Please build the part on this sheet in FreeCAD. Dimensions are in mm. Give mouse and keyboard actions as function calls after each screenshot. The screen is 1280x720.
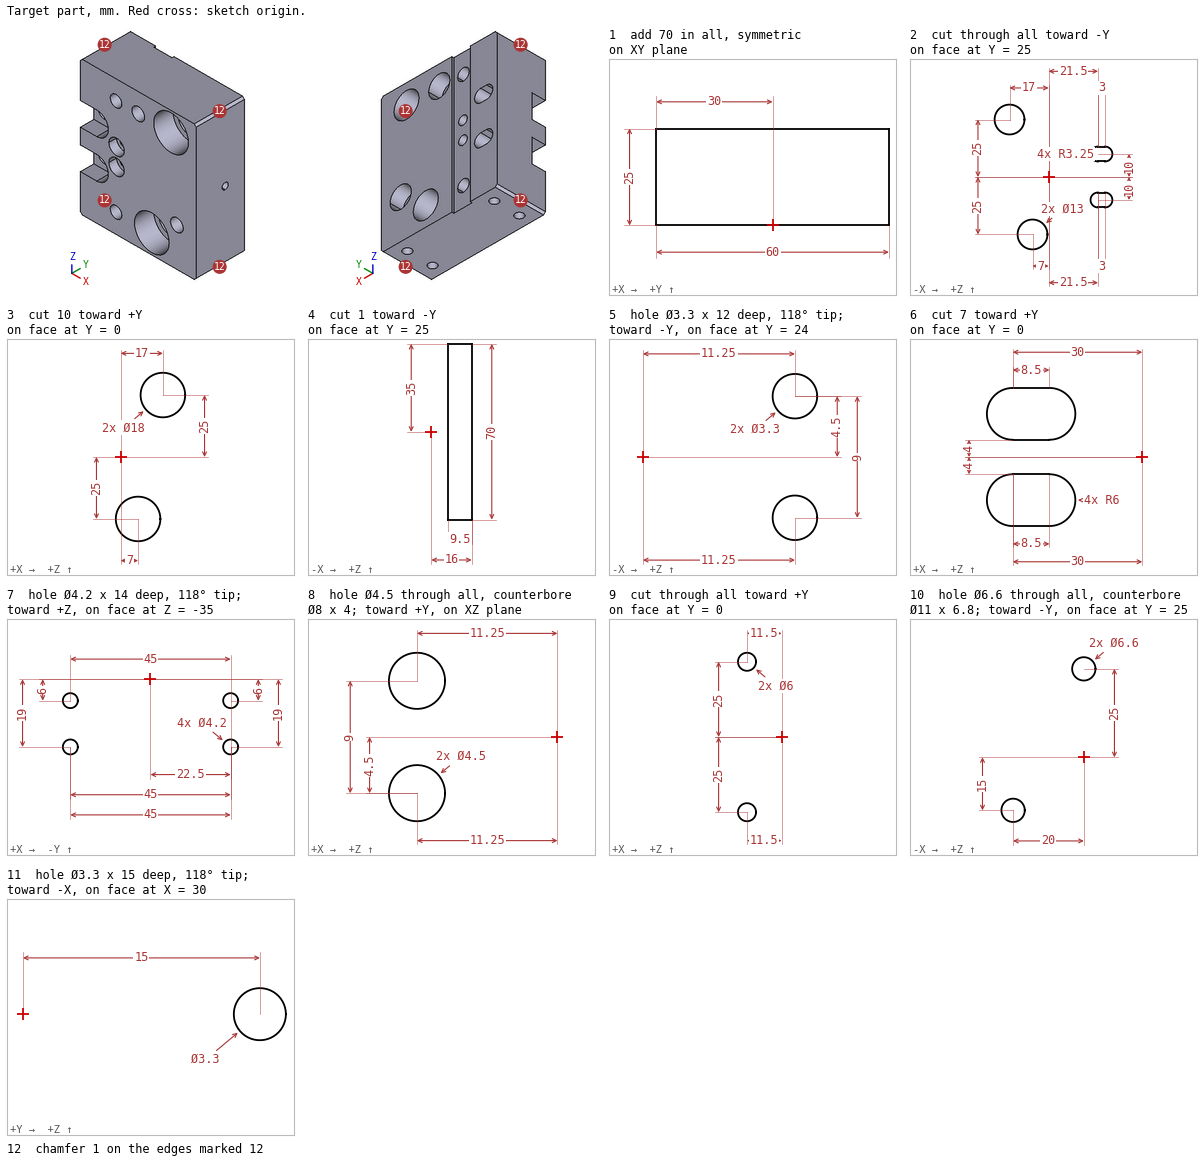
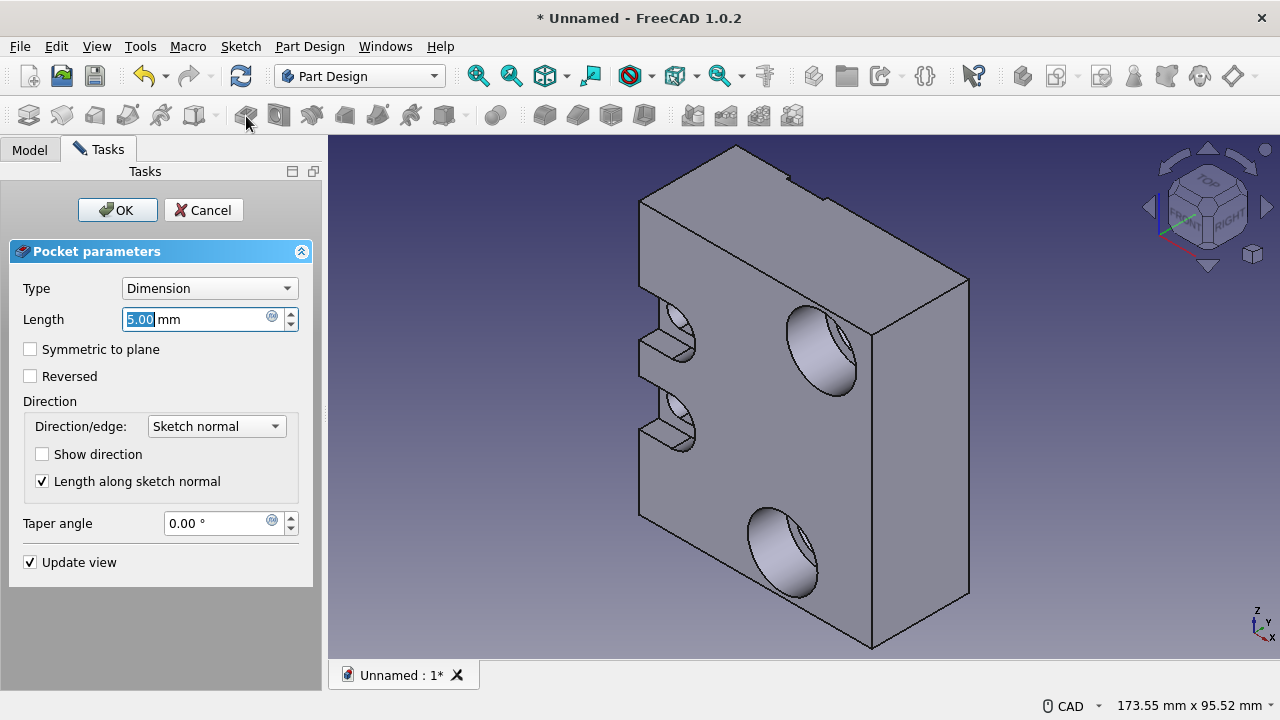
text(7)
key(Tab)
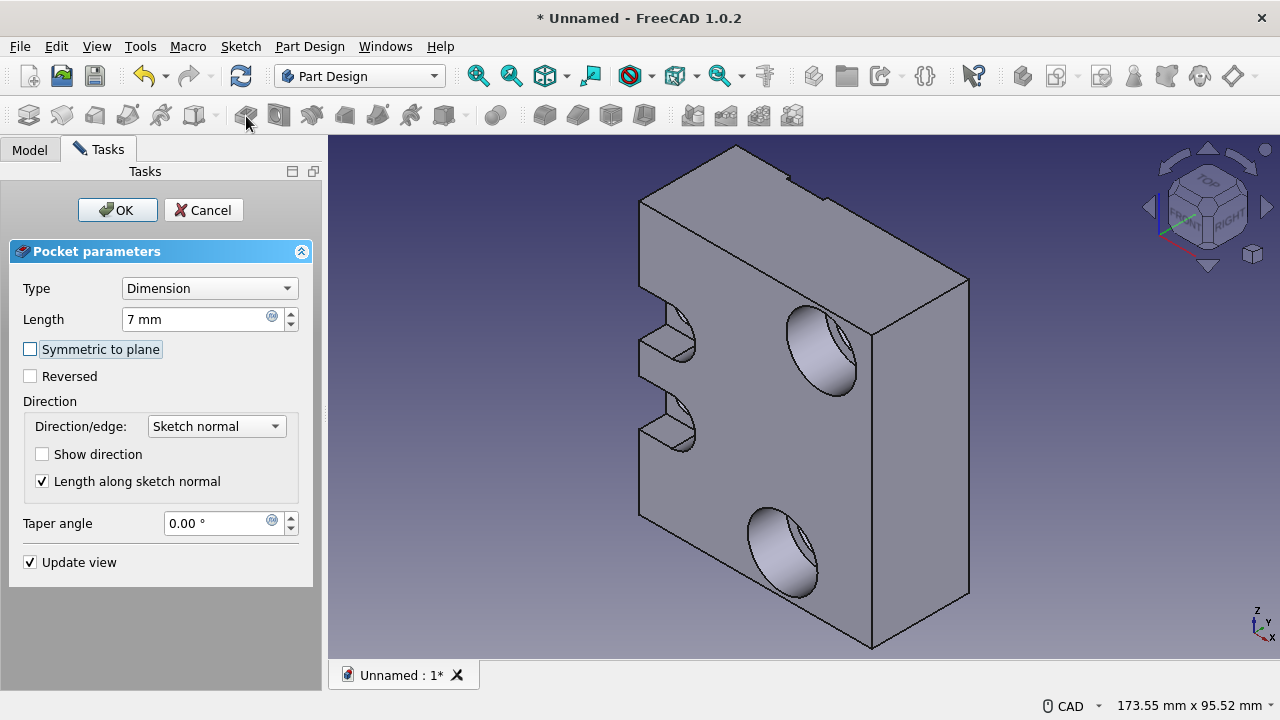
click(118, 210)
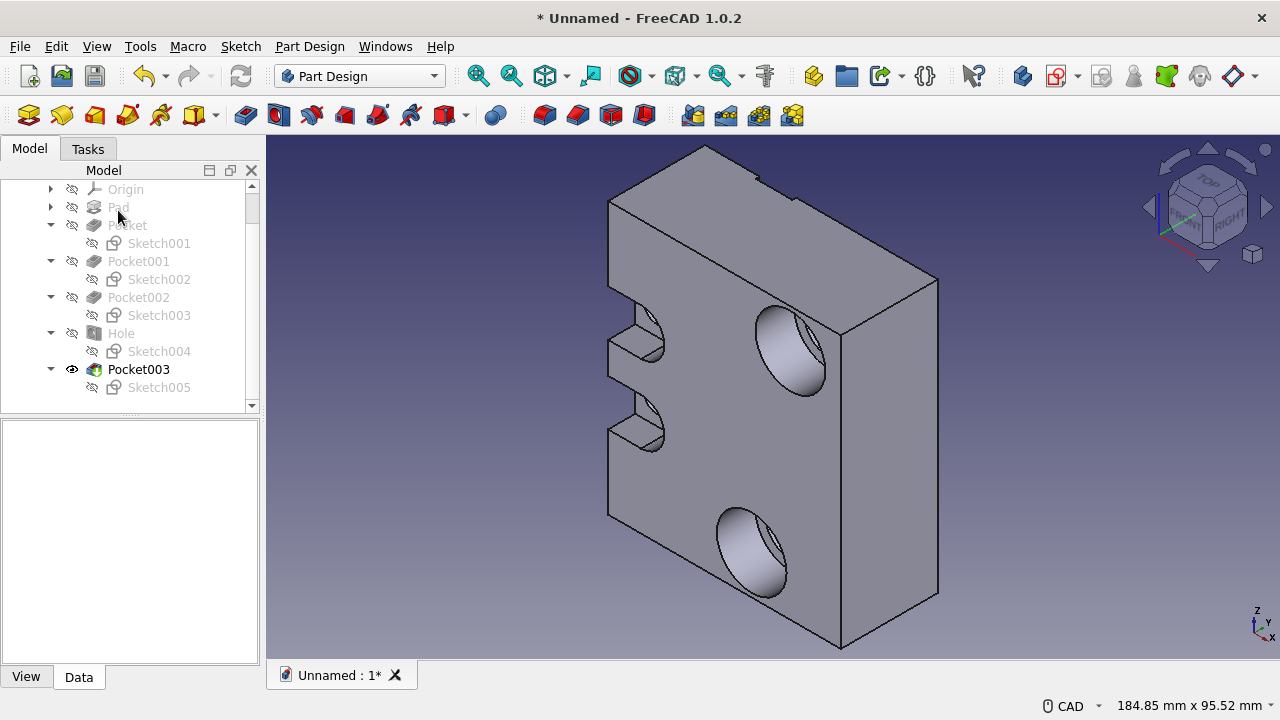
key(5)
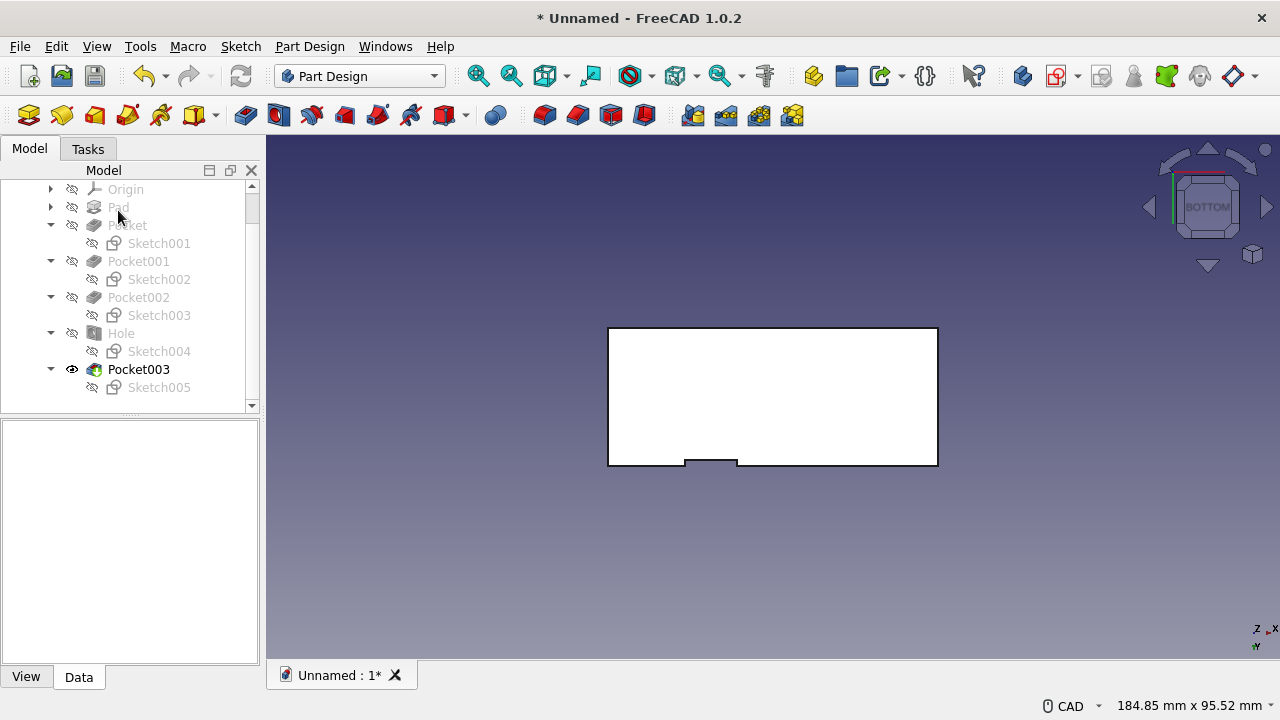
key(v)
key(f)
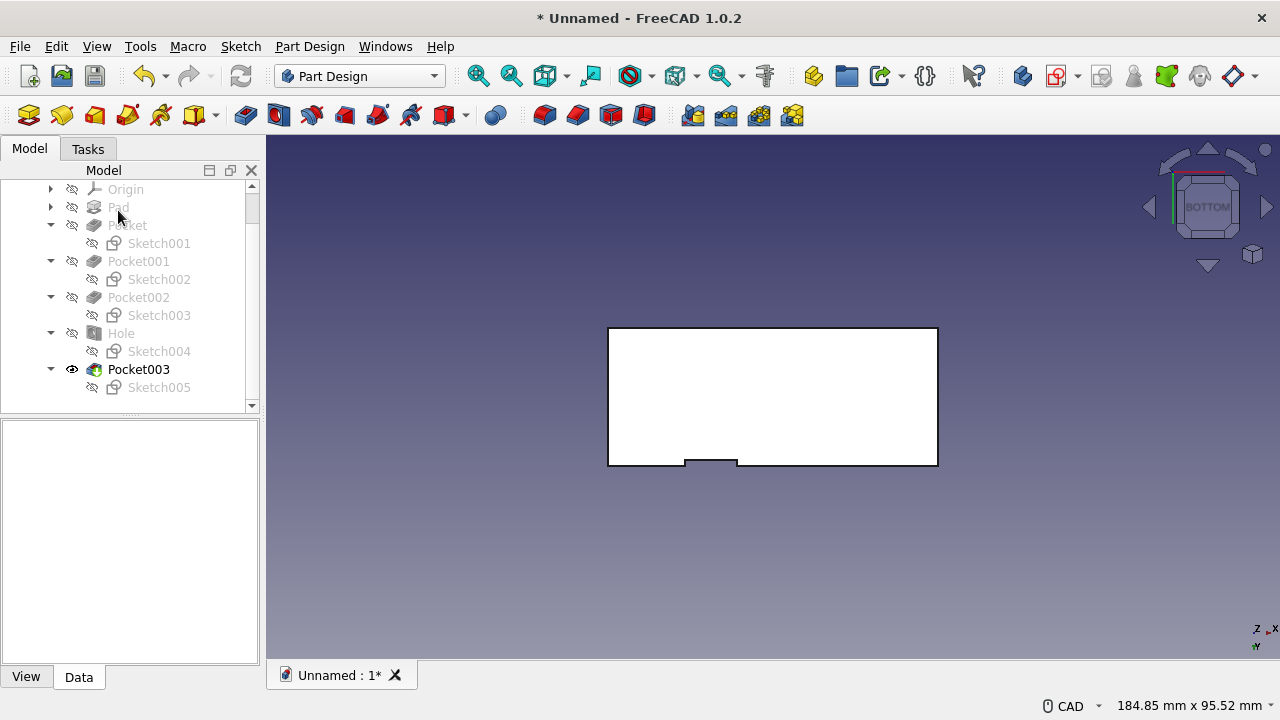
click(867, 396)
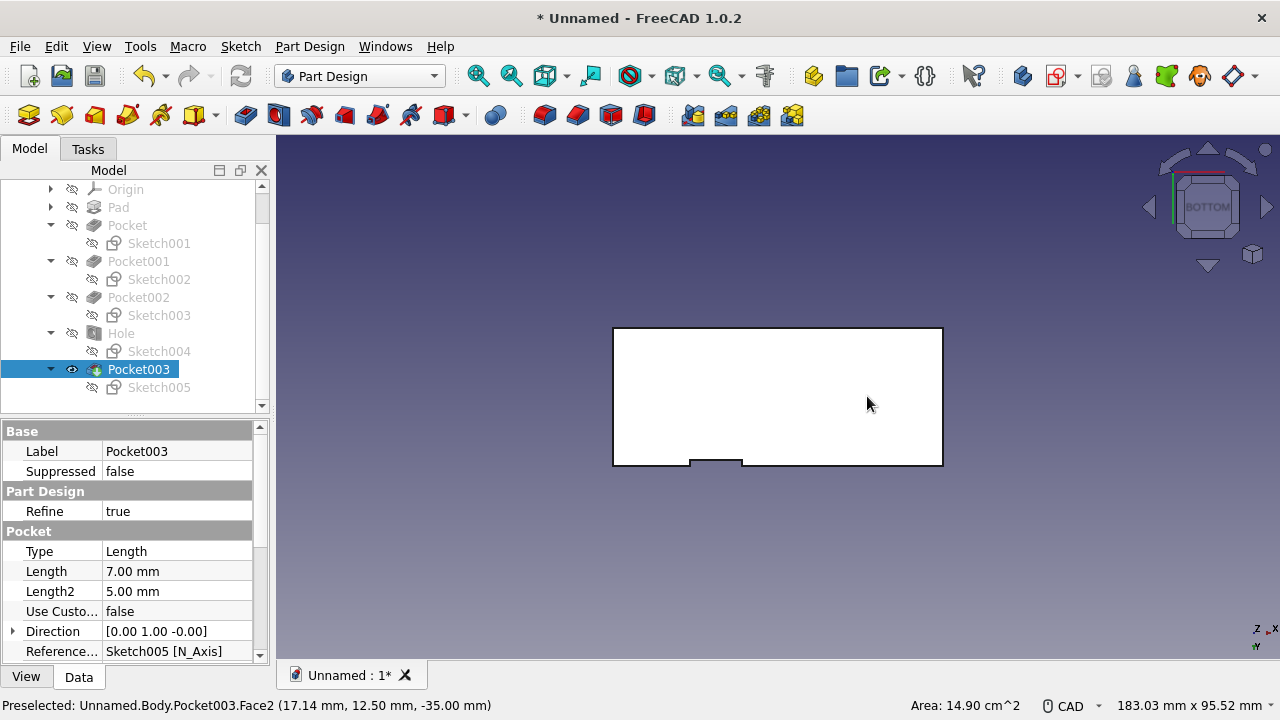
click(1056, 76)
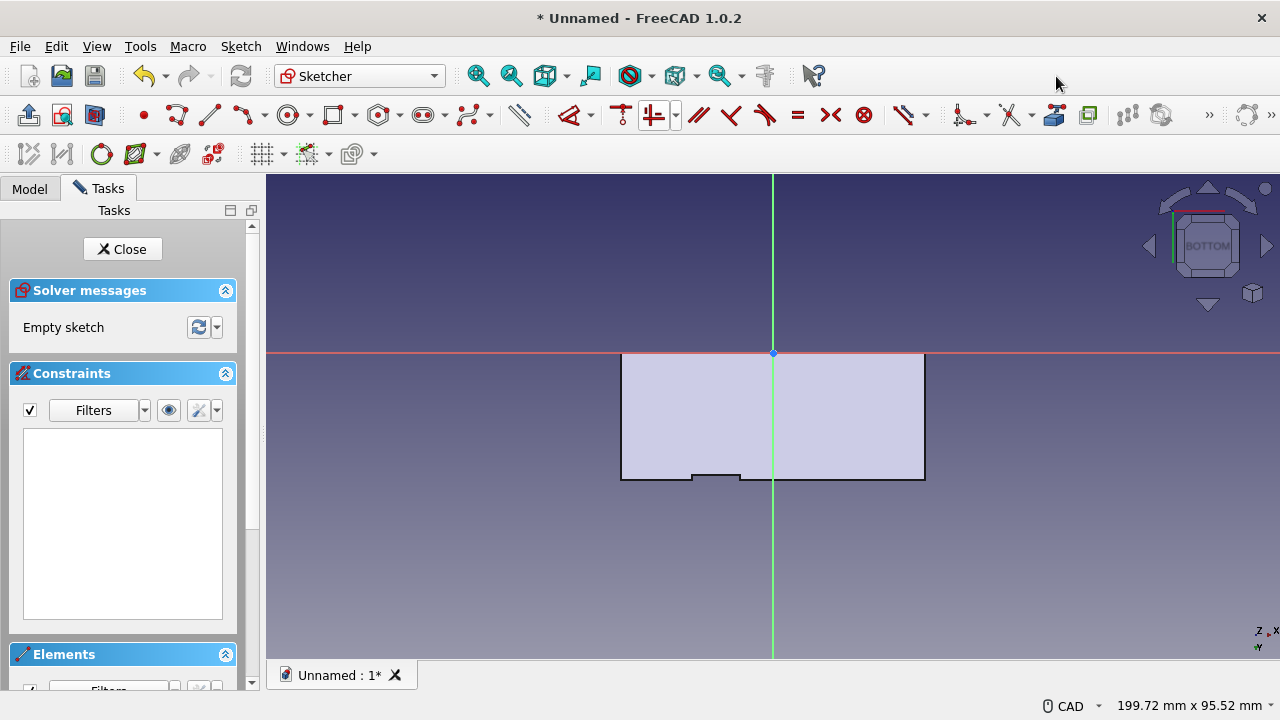
scroll(829, 399, up, 4)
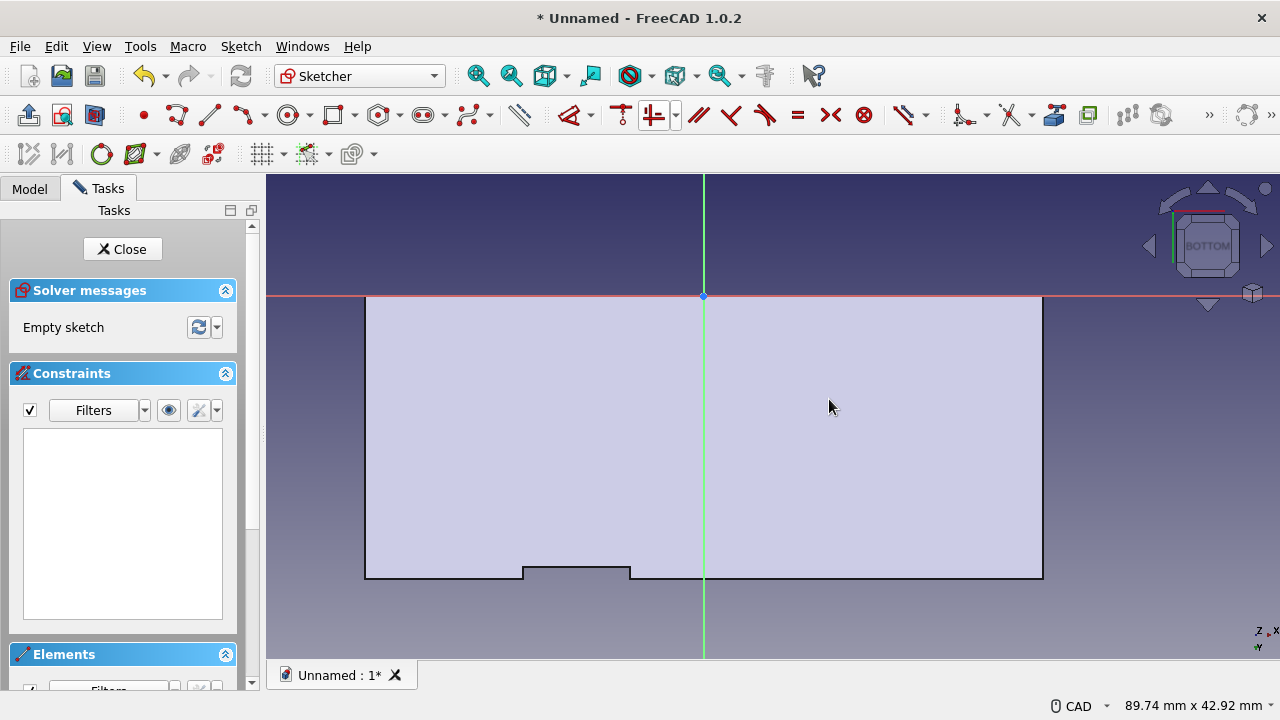
key(g)
key(c)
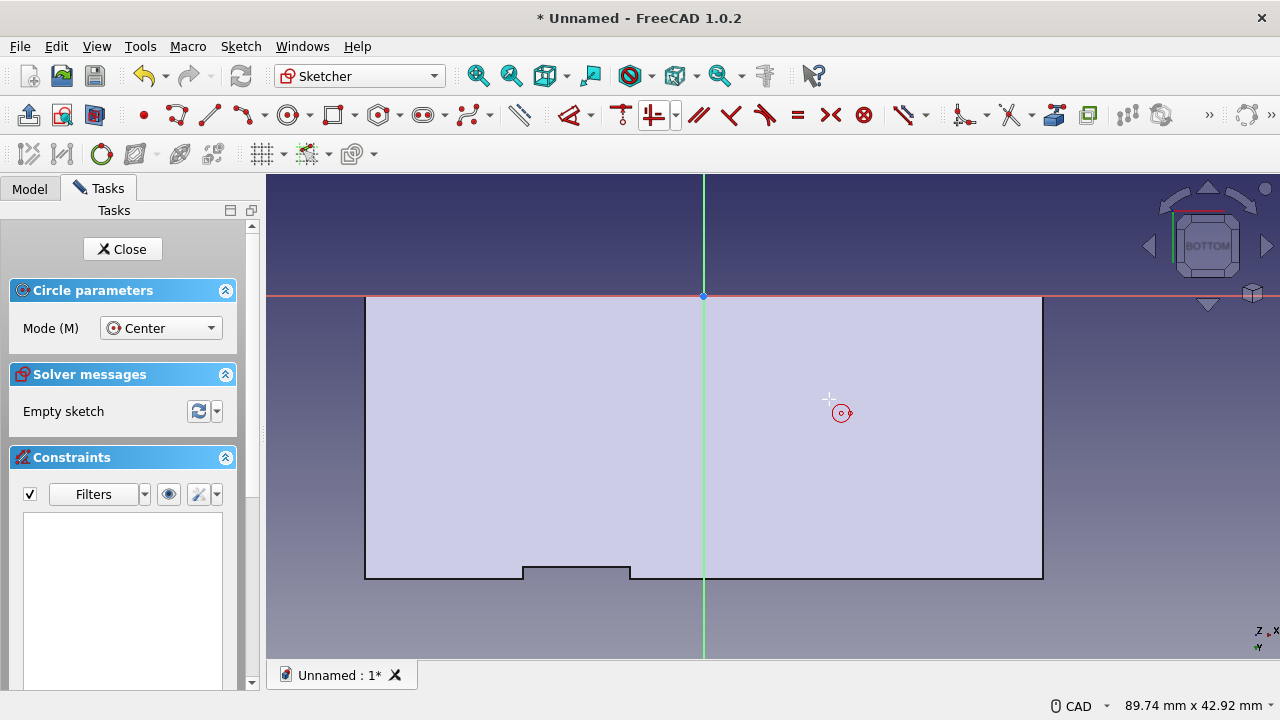
click(958, 511)
move(975, 494)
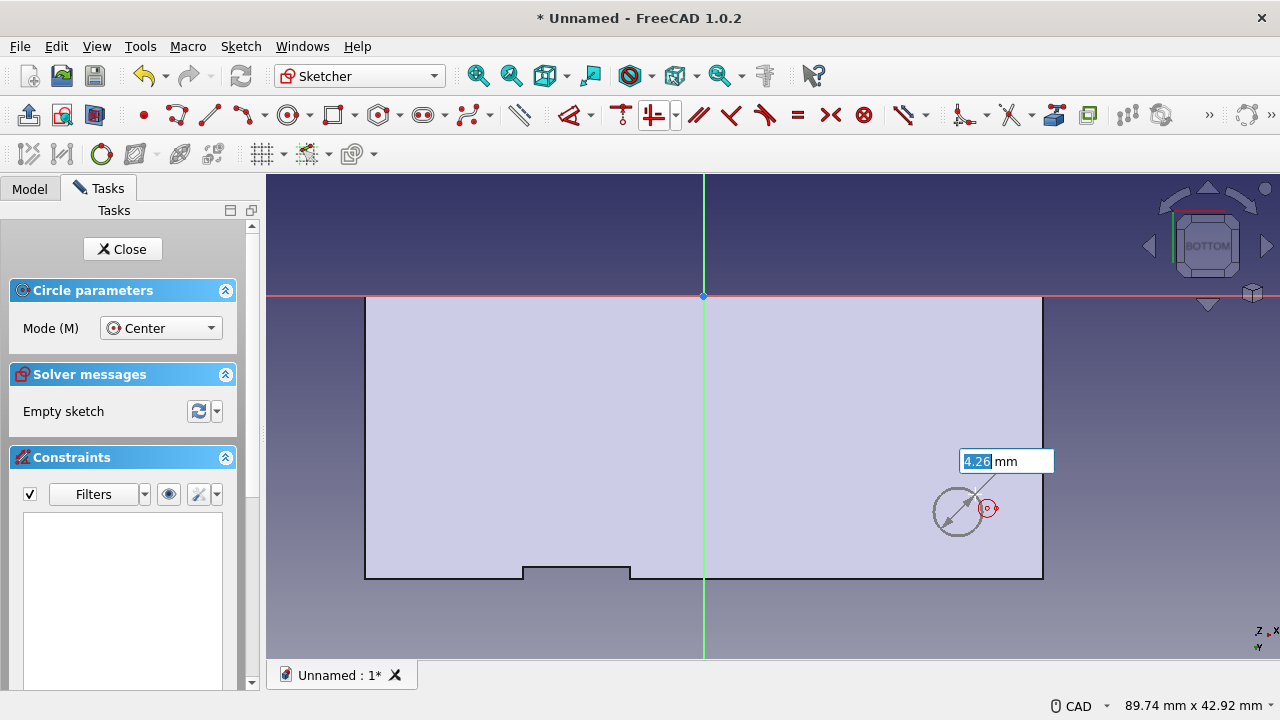
text(4.2)
key(Return)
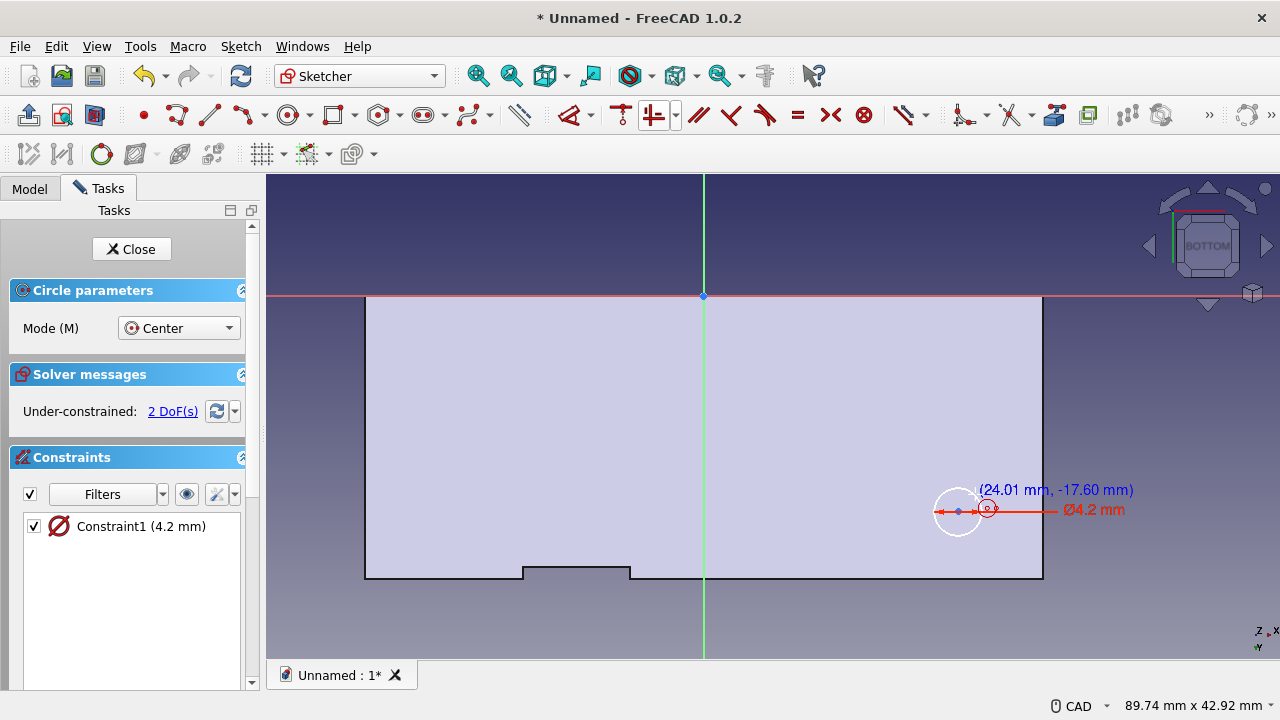
click(958, 364)
move(975, 347)